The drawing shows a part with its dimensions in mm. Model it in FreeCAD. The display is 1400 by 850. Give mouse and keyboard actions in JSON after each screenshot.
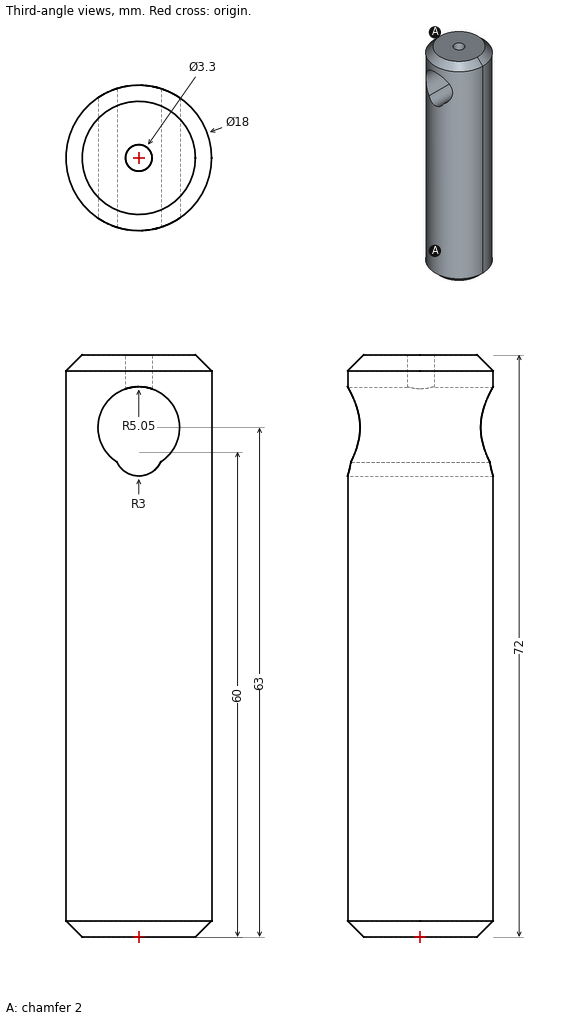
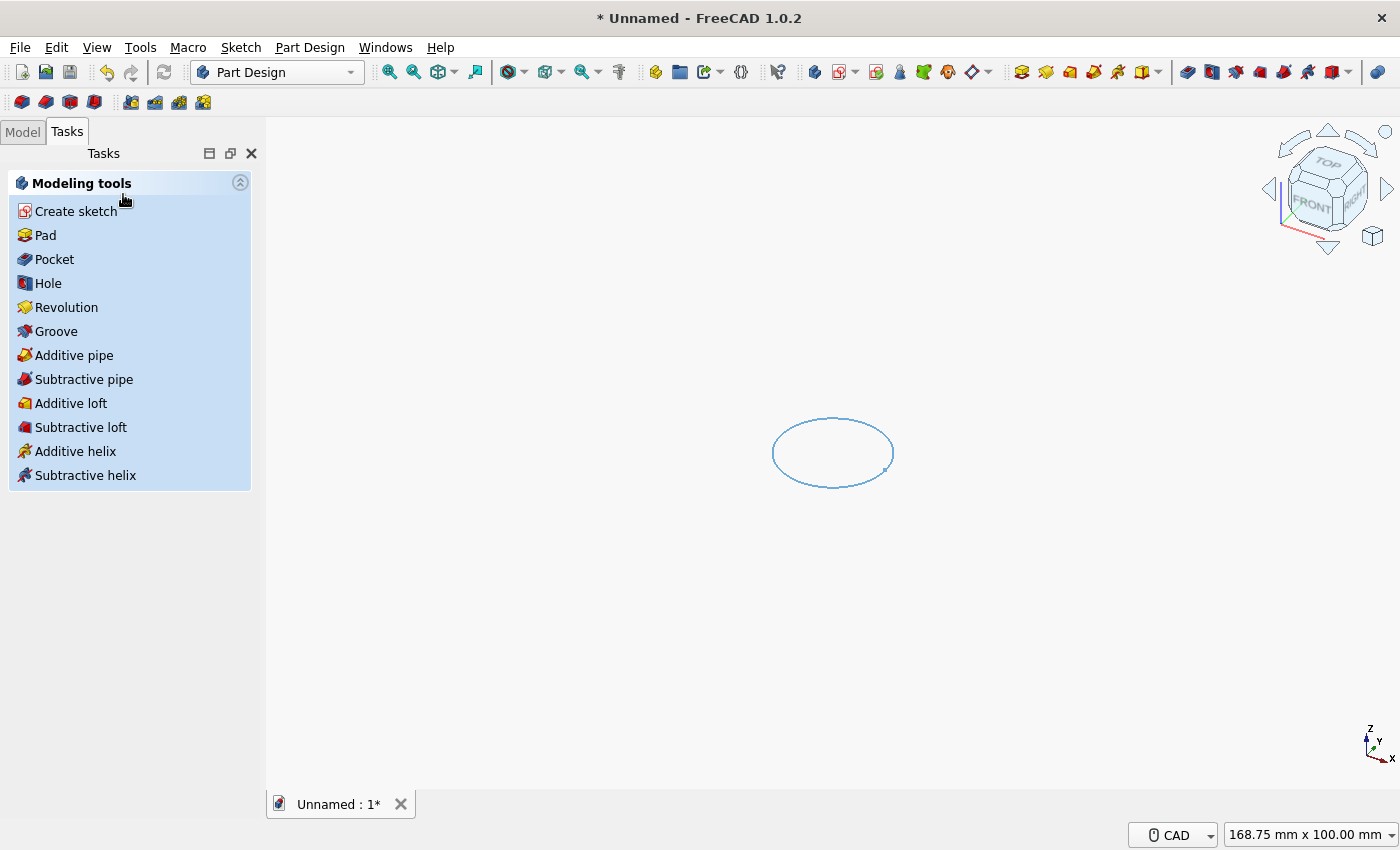
{"action": "left_click", "coordinate": [1022, 72]}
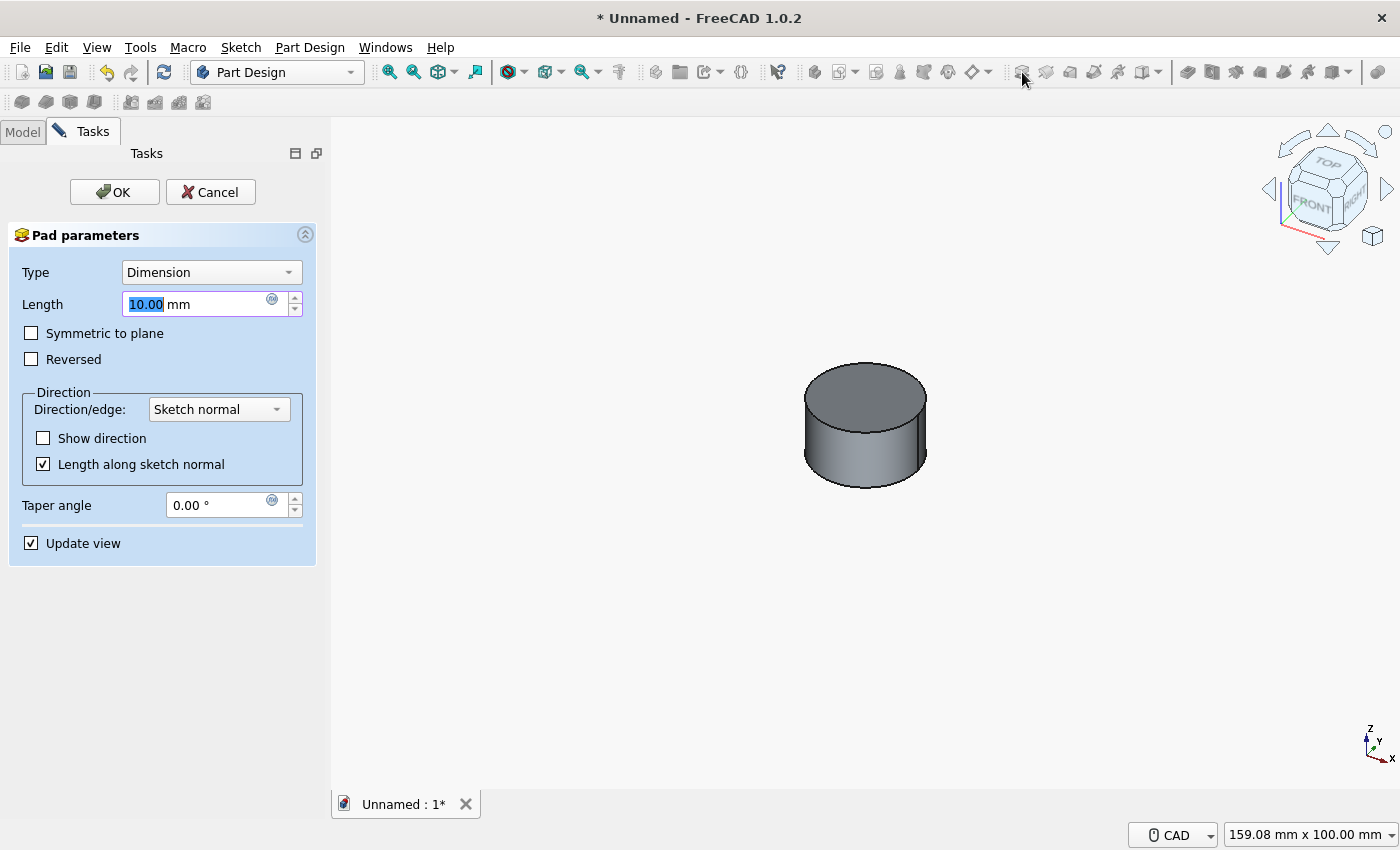
{"action": "type", "text": "72"}
{"action": "key", "text": "Tab"}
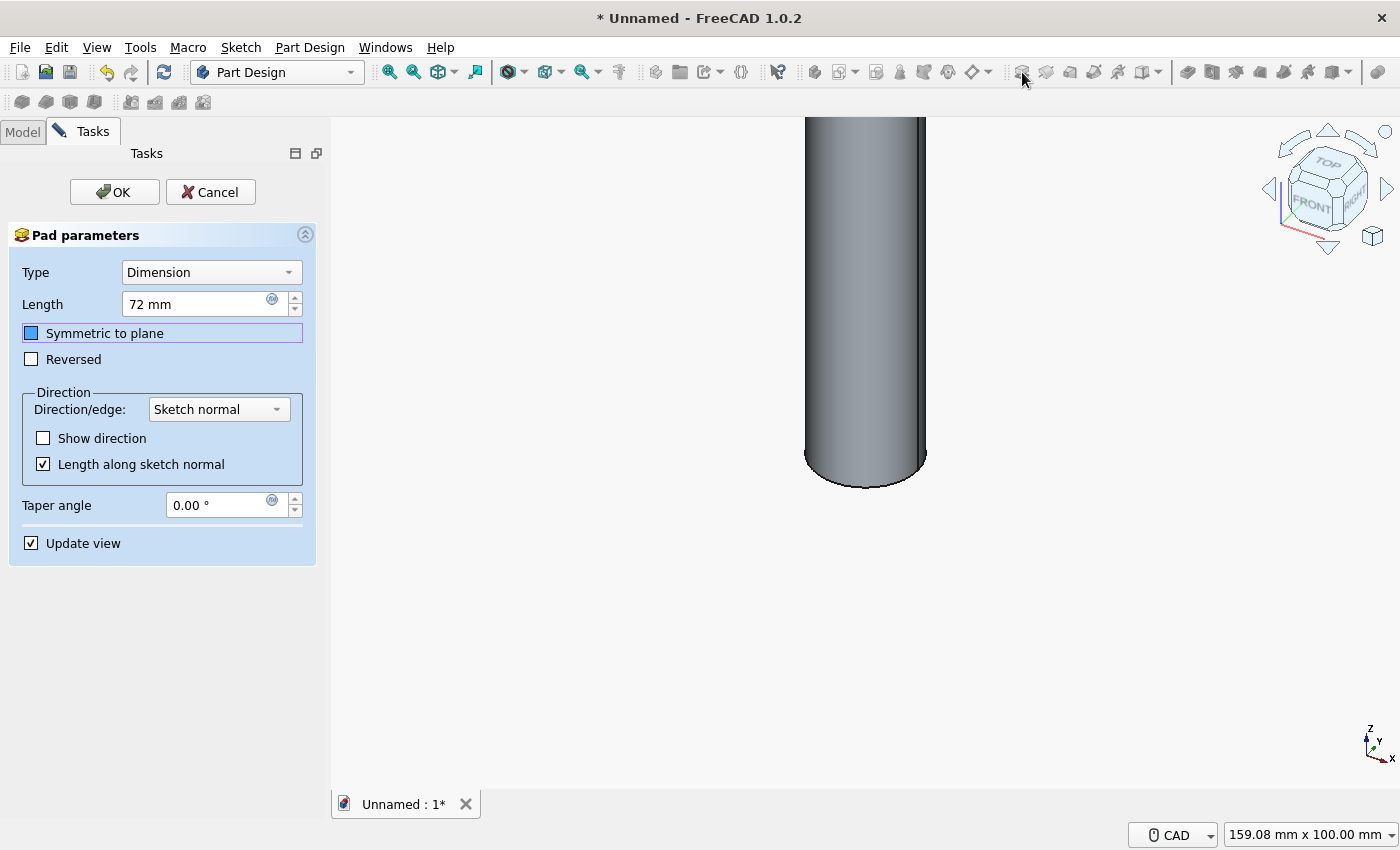
{"action": "left_click", "coordinate": [115, 192]}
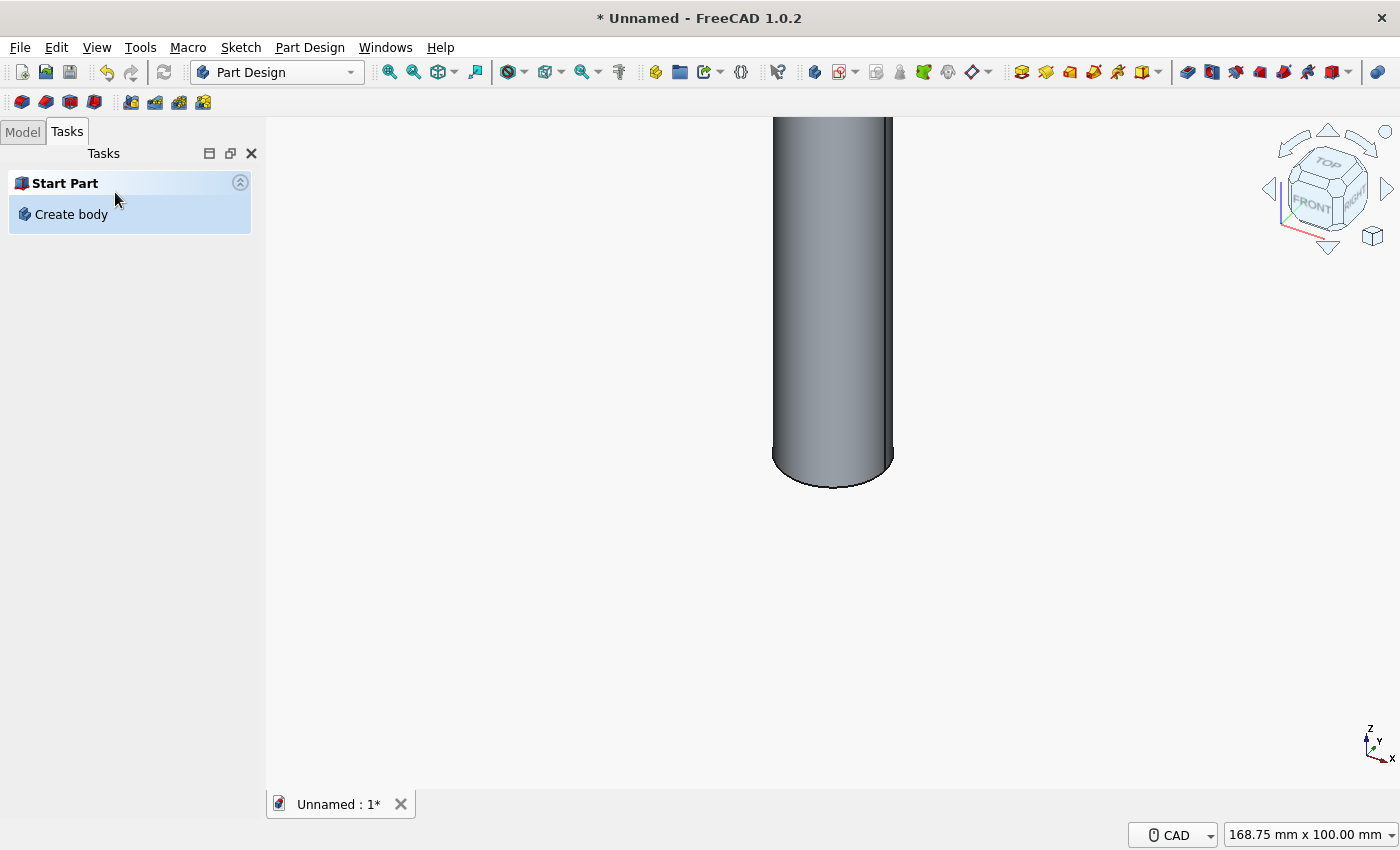
{"action": "left_click", "coordinate": [390, 72]}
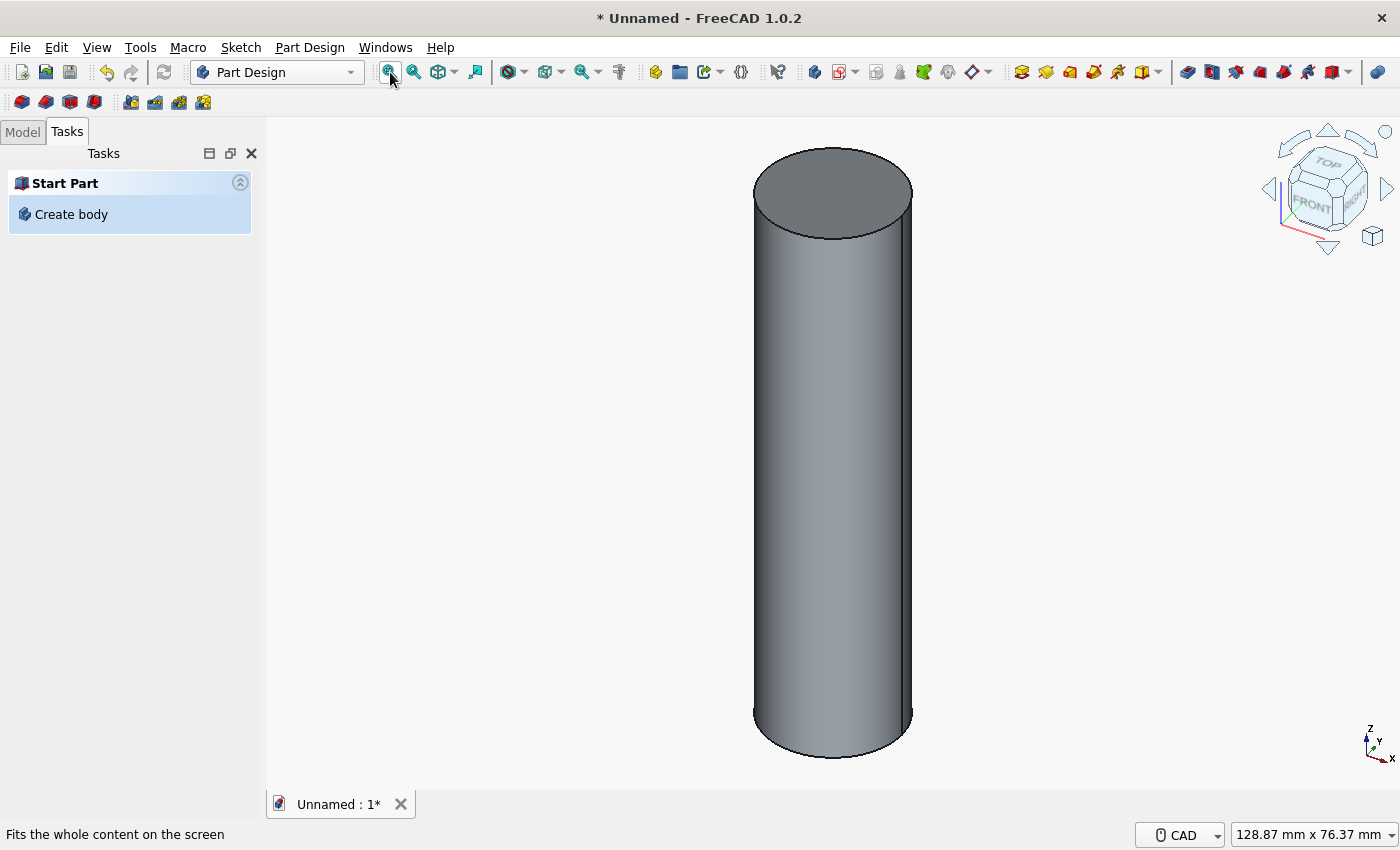
{"action": "left_click", "coordinate": [840, 72]}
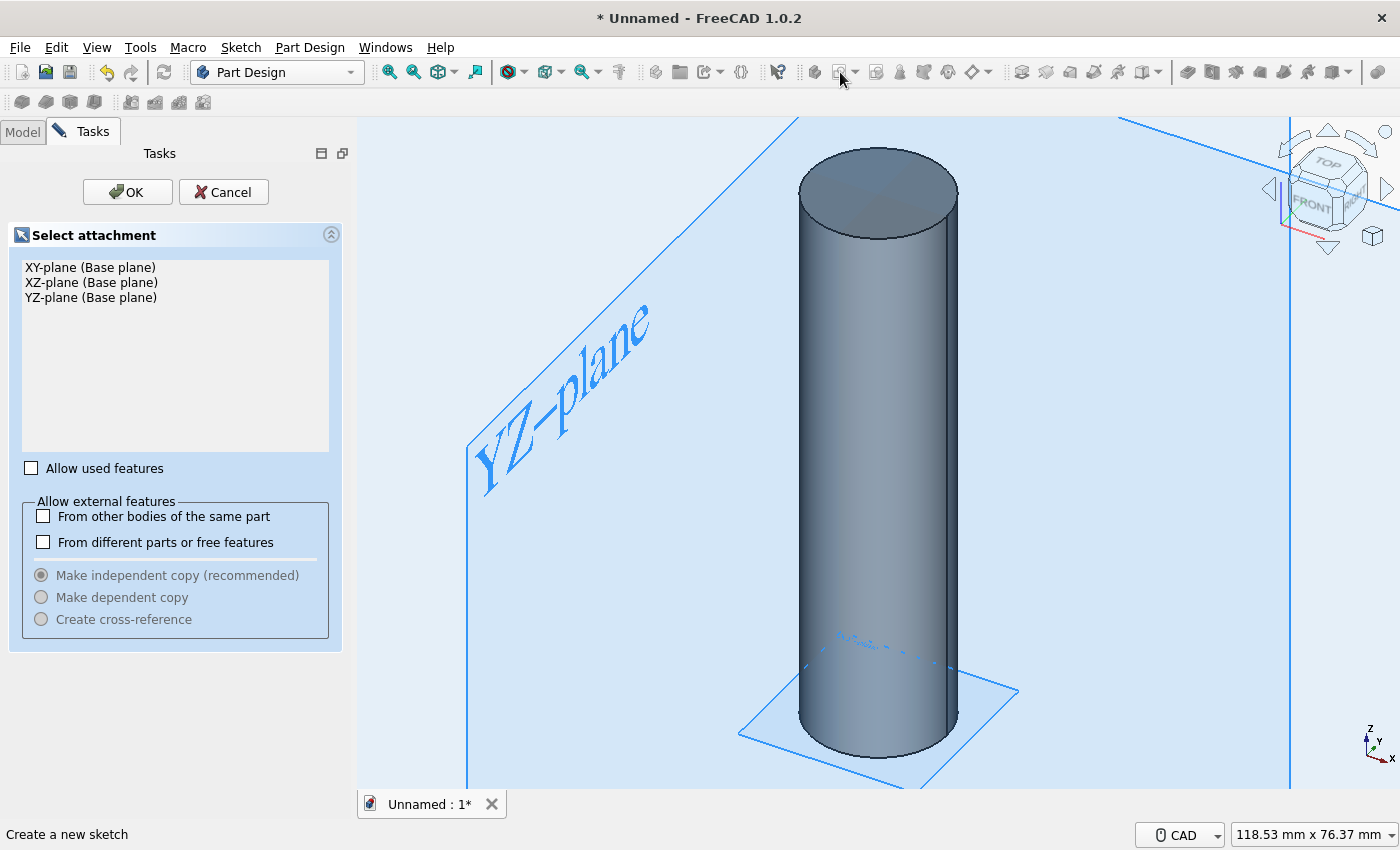
{"action": "left_click", "coordinate": [82, 282]}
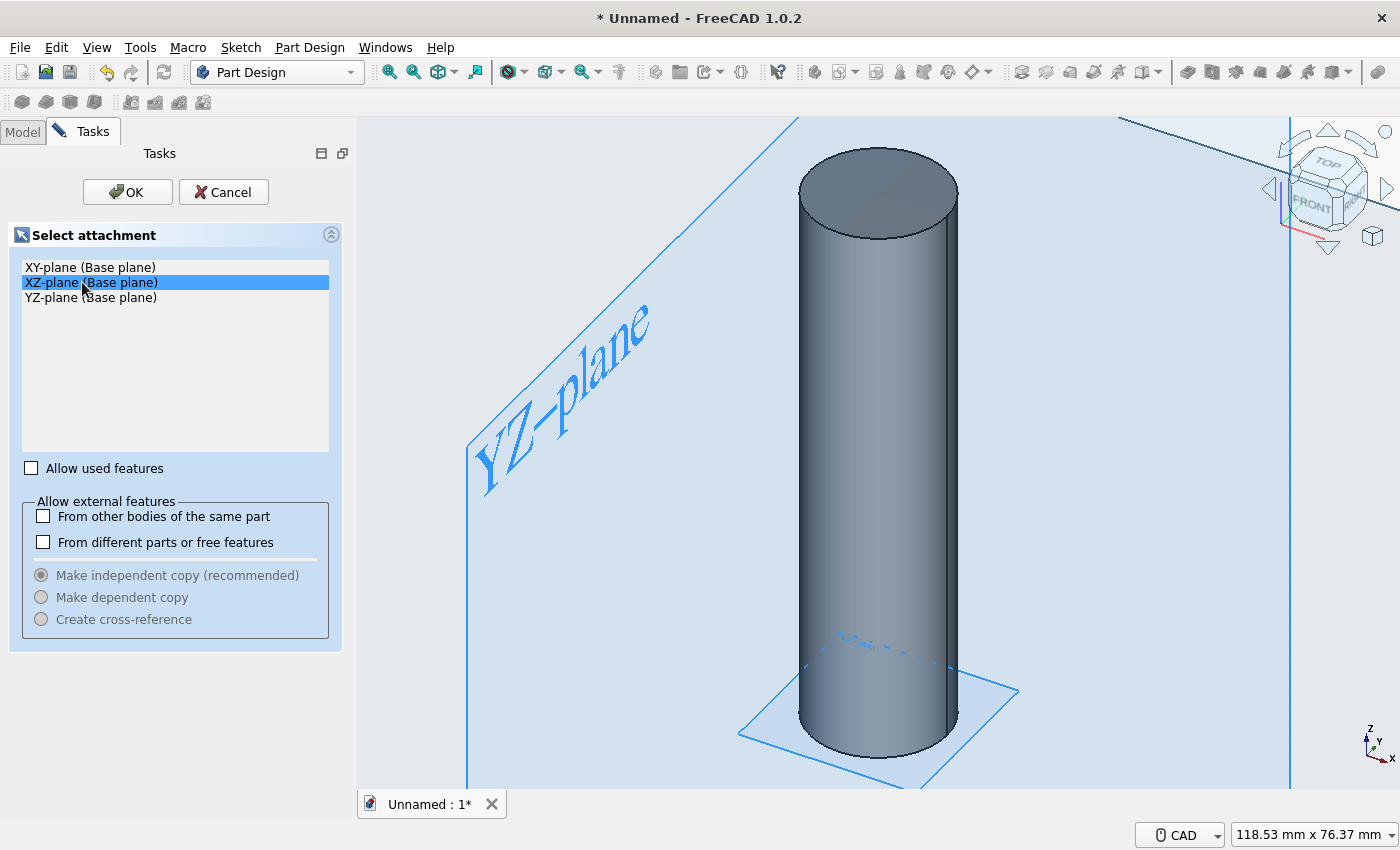
{"action": "left_click", "coordinate": [128, 192]}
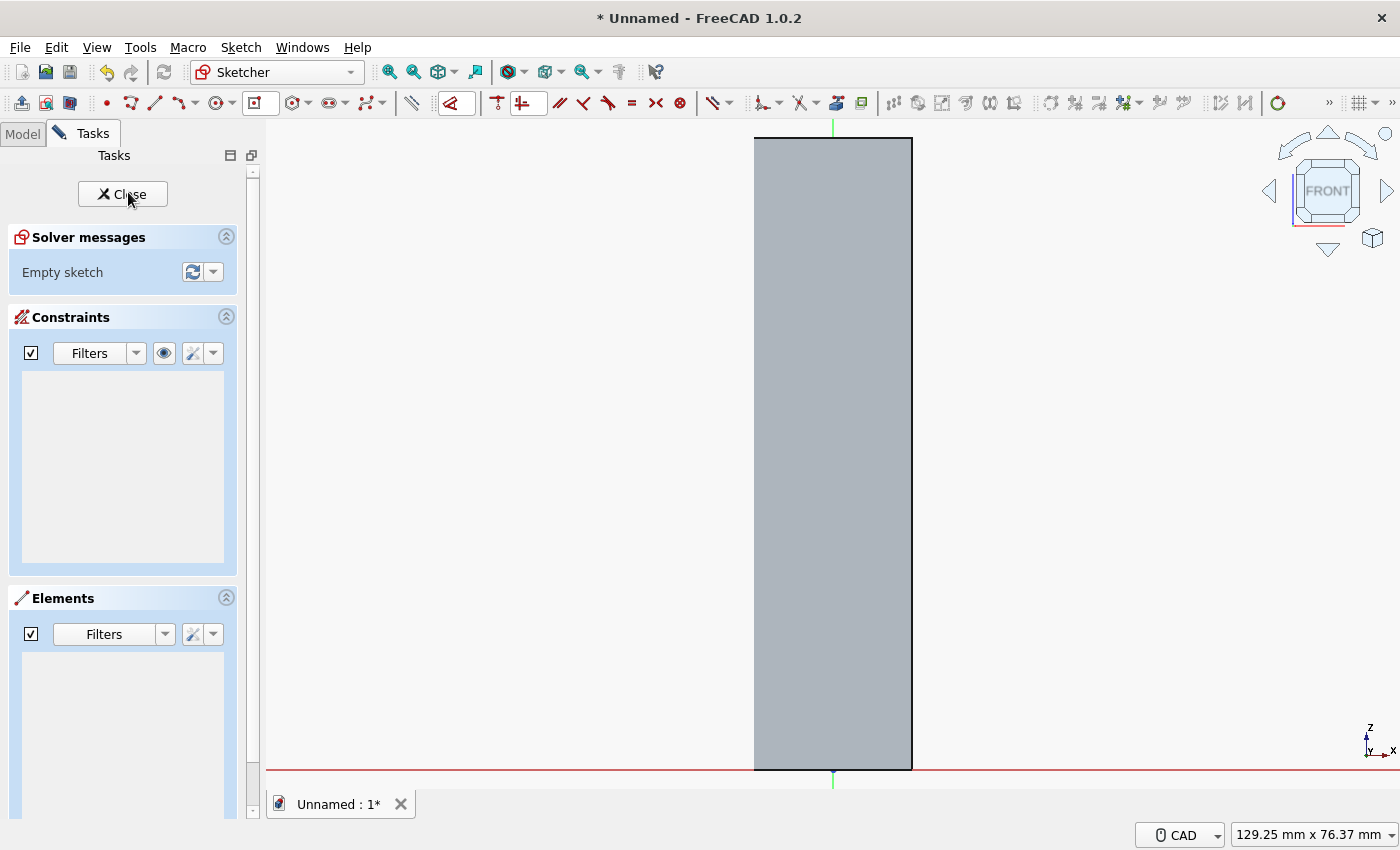
{"action": "key", "text": "q s"}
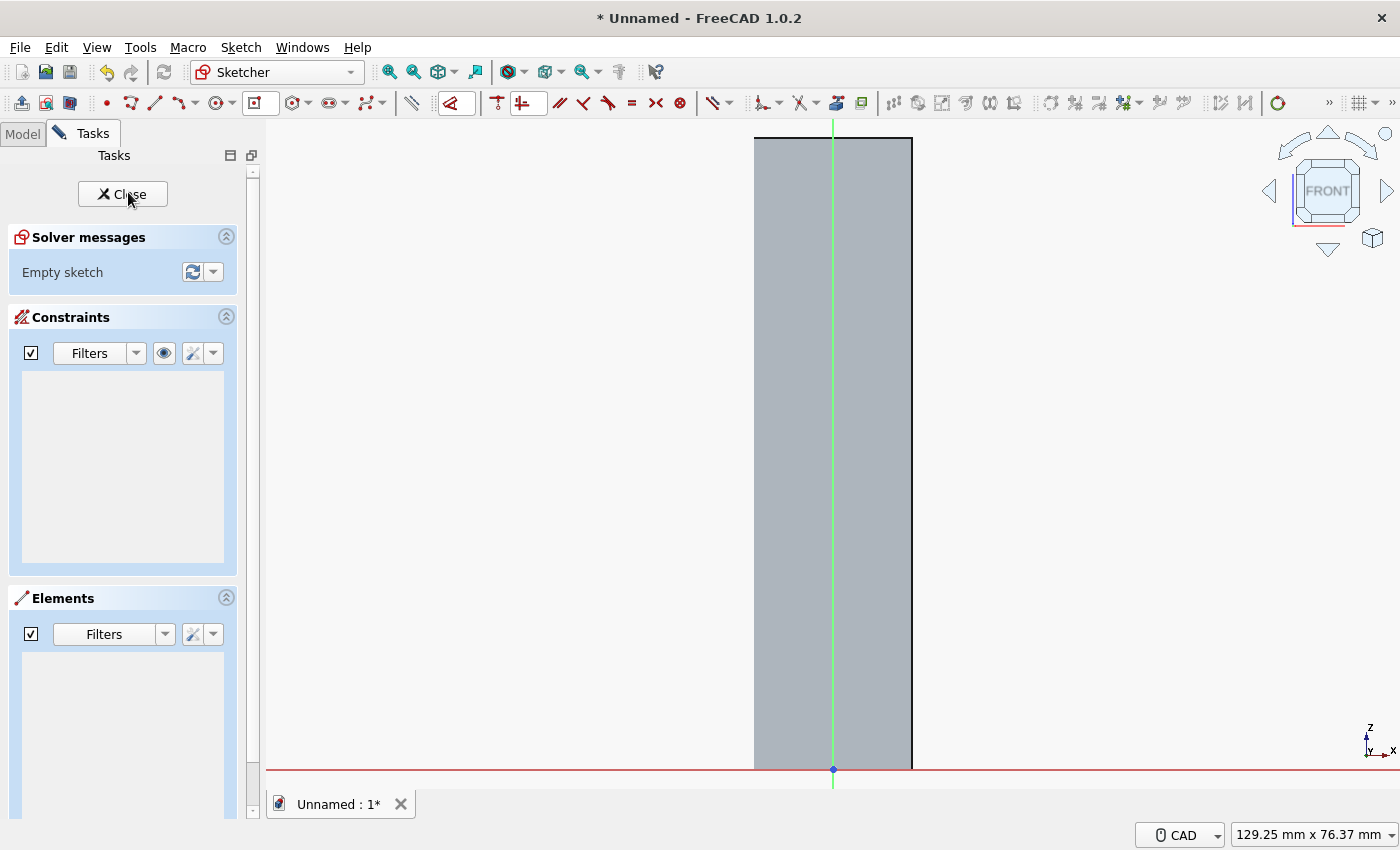
{"action": "scroll", "coordinate": [855, 147], "scroll_direction": "up", "scroll_amount": 7}